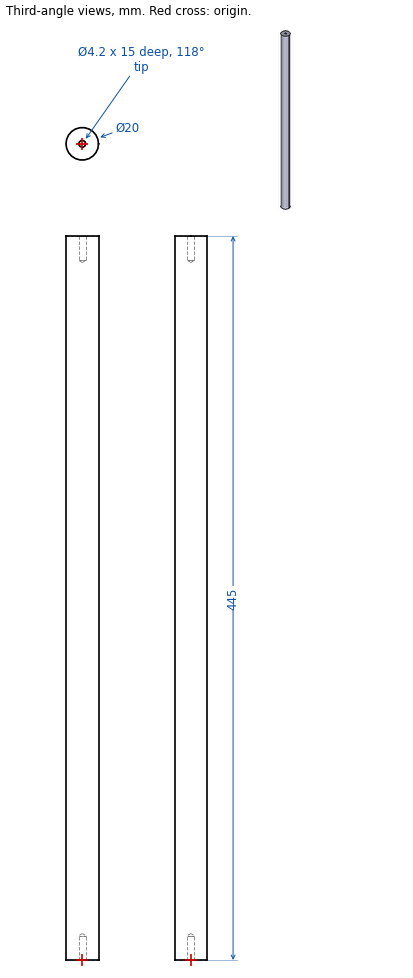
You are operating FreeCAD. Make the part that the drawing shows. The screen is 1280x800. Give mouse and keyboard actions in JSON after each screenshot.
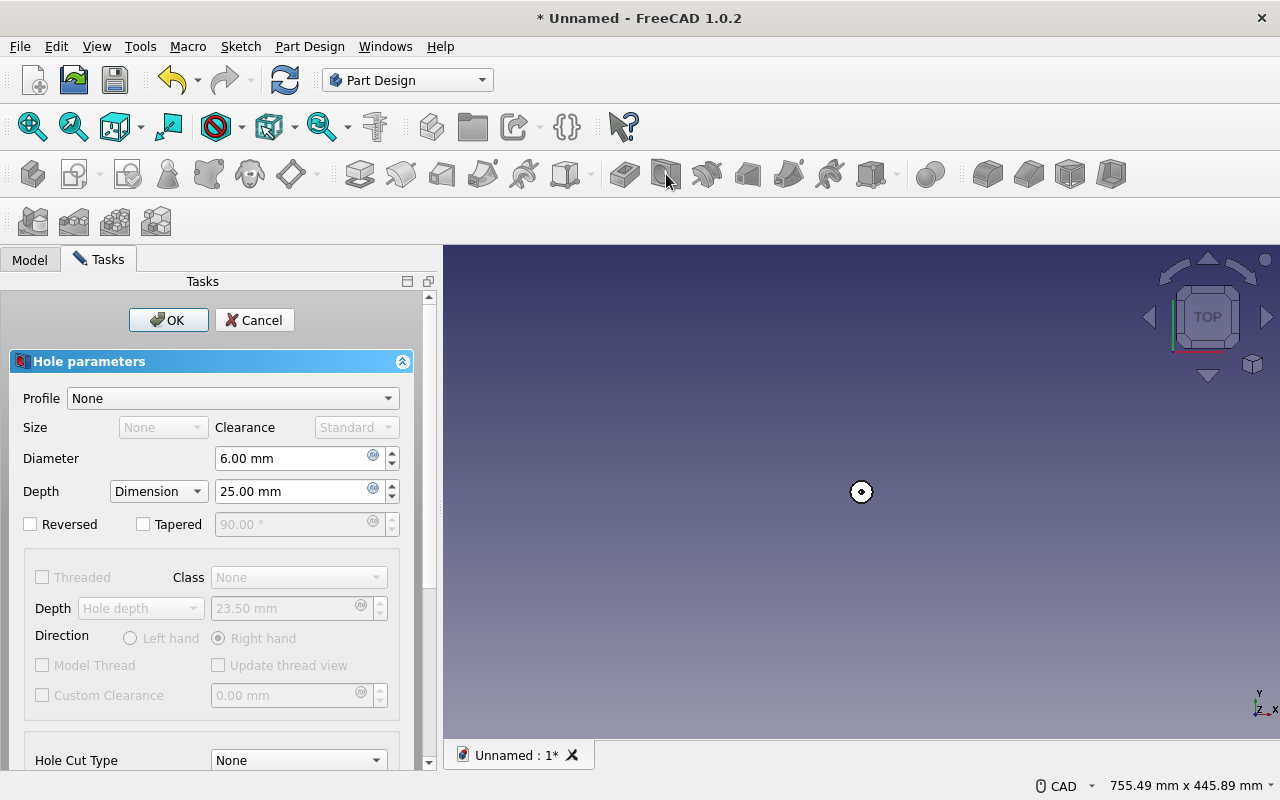
{"action": "triple_click", "coordinate": [300, 458]}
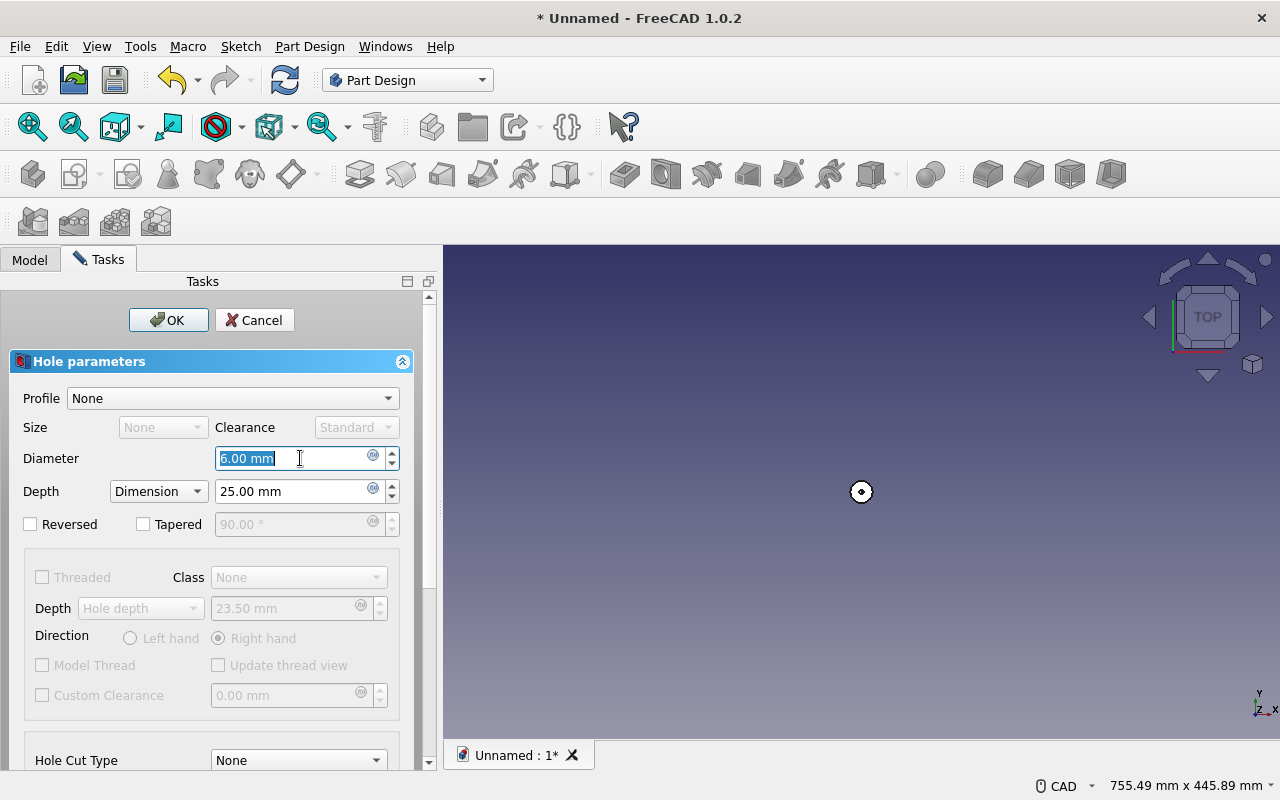
{"action": "type", "text": "4.2"}
{"action": "key", "text": "Tab"}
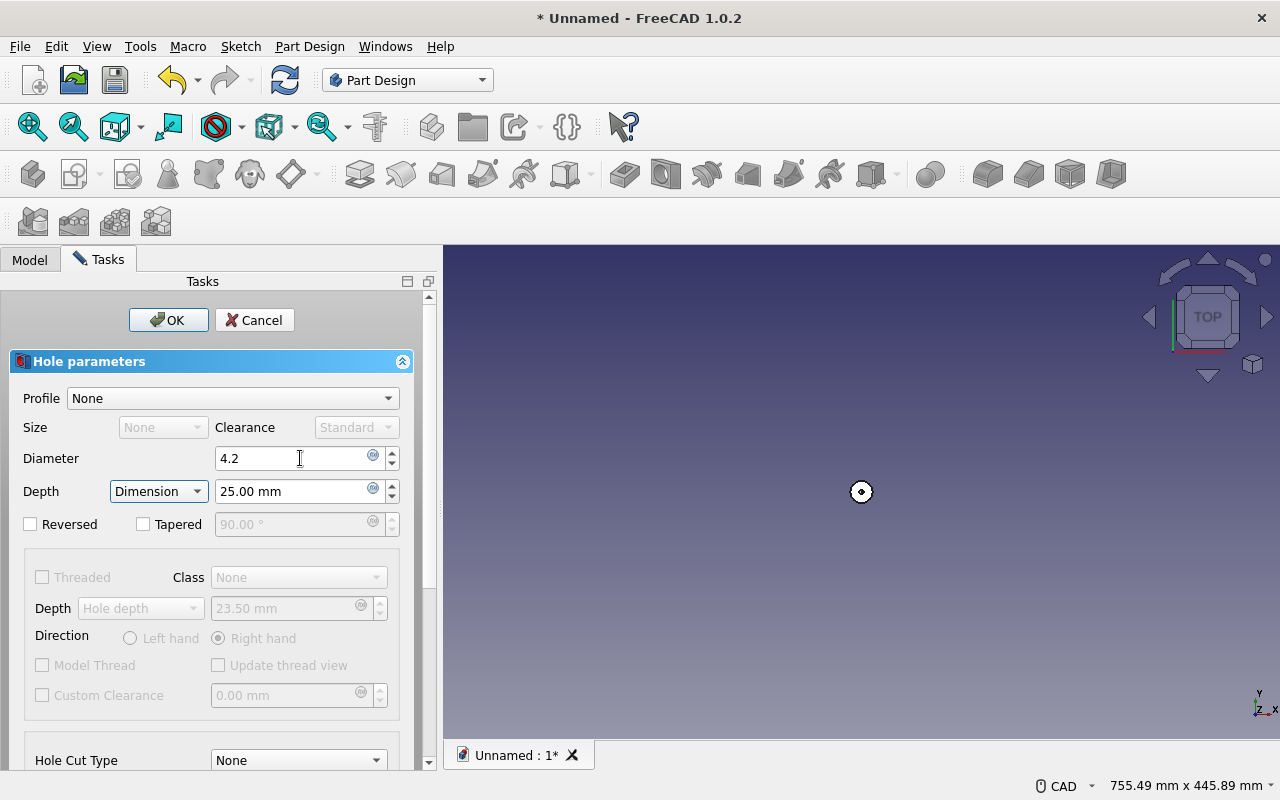
{"action": "triple_click", "coordinate": [300, 492]}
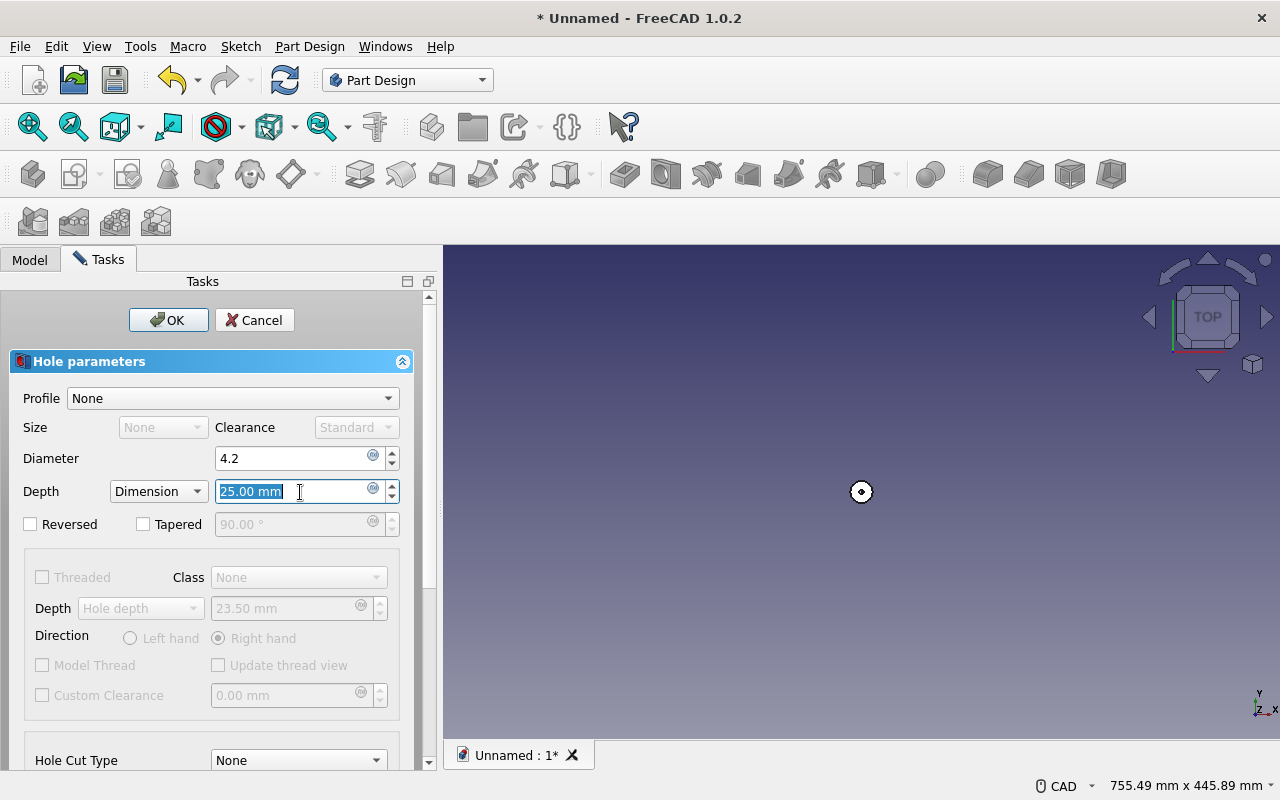
{"action": "type", "text": "15"}
{"action": "key", "text": "Tab"}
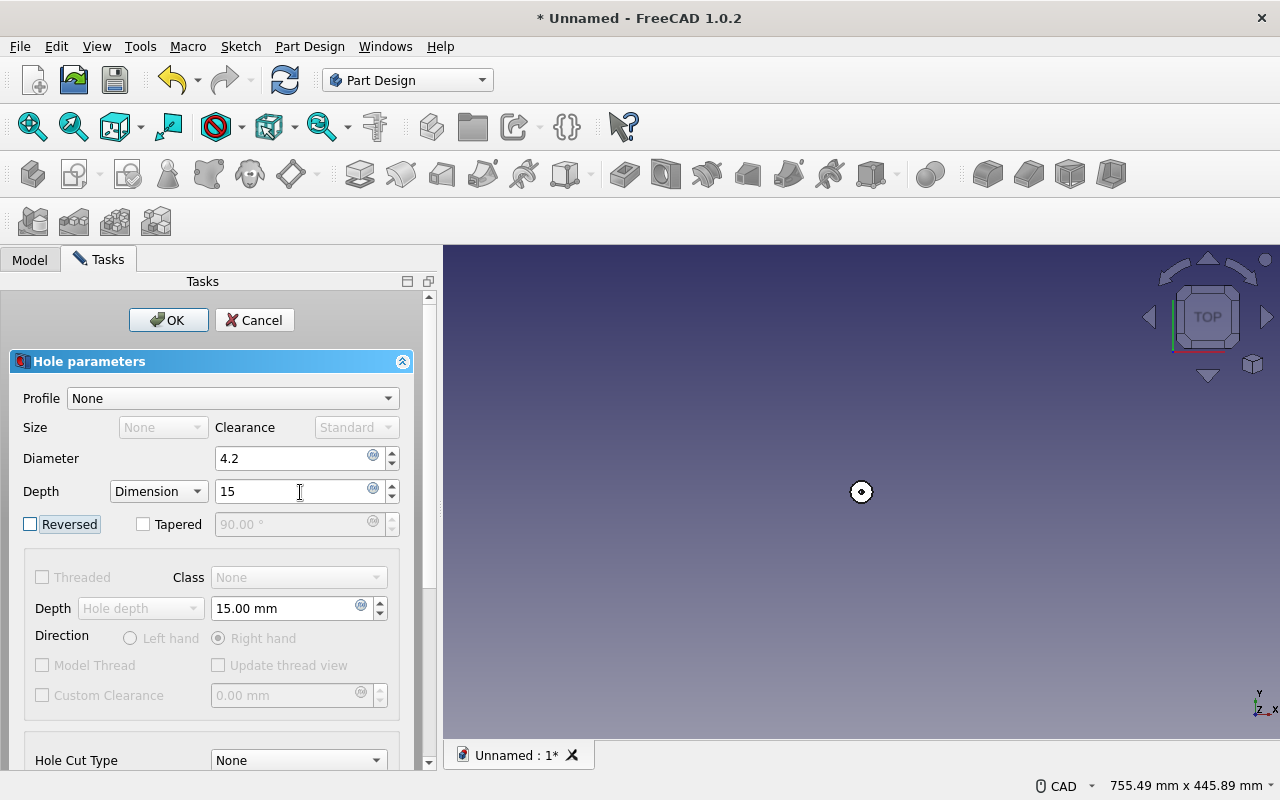
{"action": "left_click", "coordinate": [31, 524]}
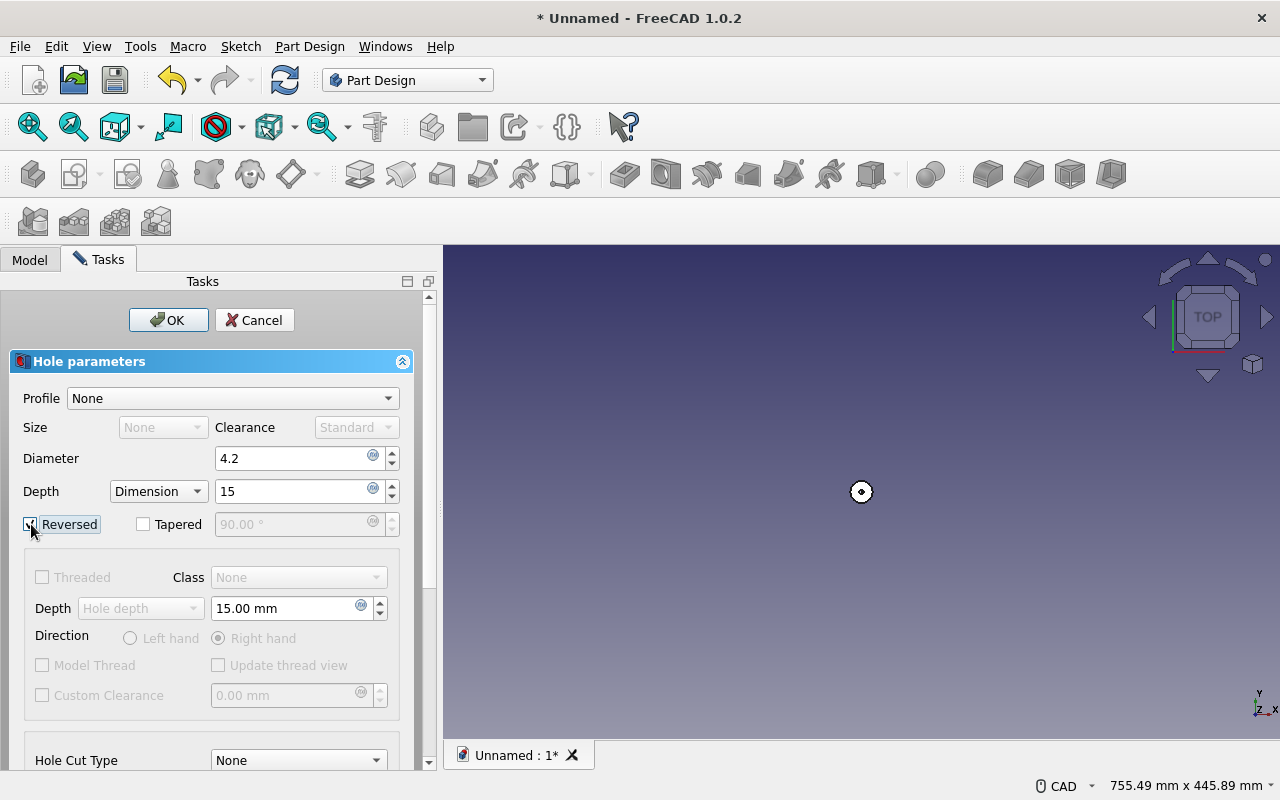
{"action": "left_click", "coordinate": [169, 320]}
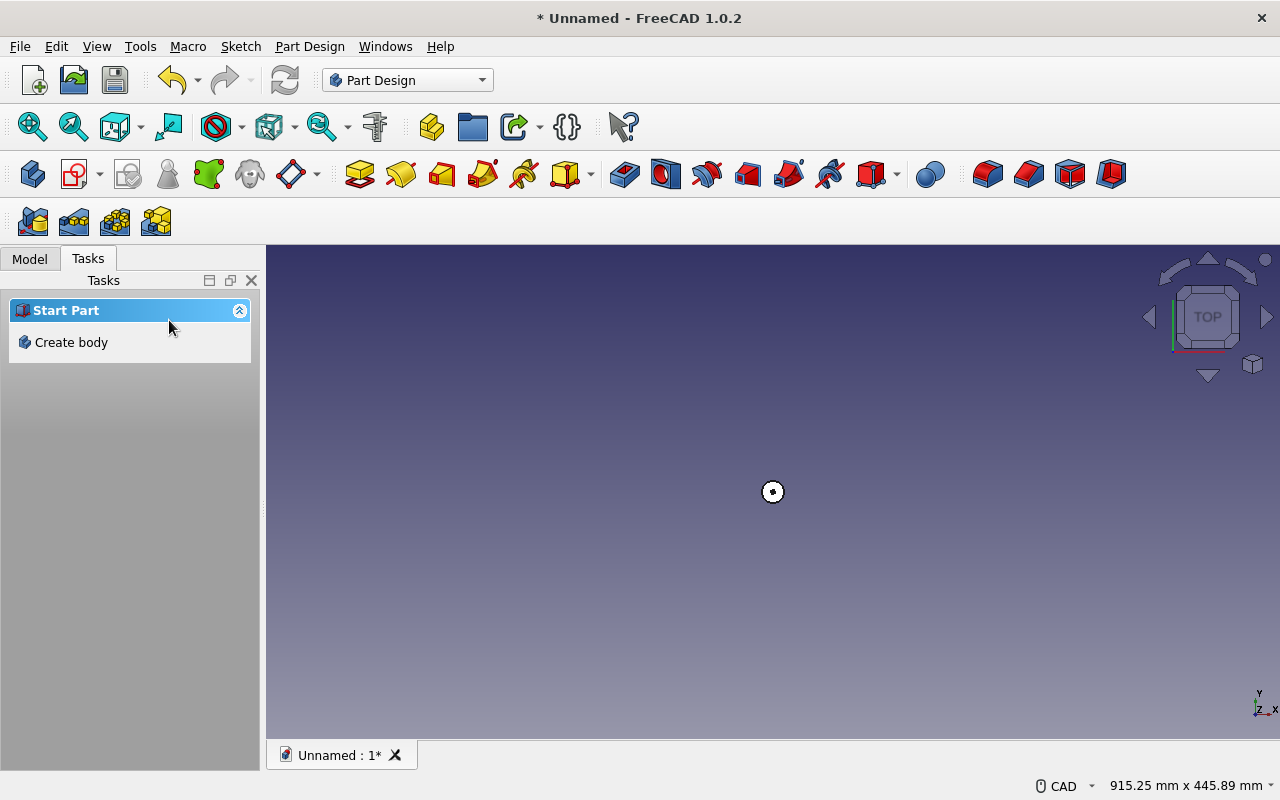
{"action": "key", "text": "0"}